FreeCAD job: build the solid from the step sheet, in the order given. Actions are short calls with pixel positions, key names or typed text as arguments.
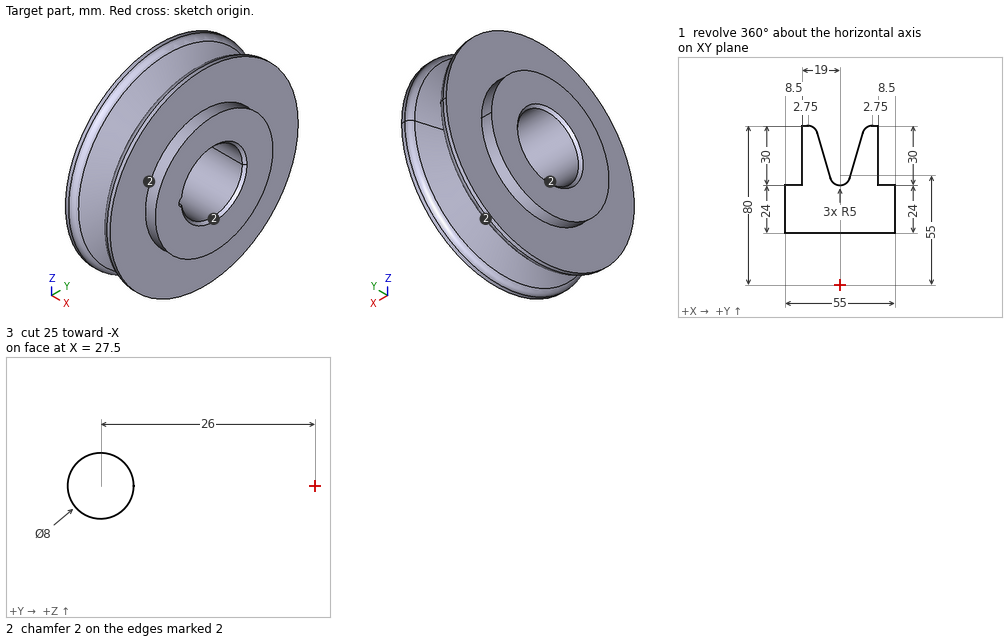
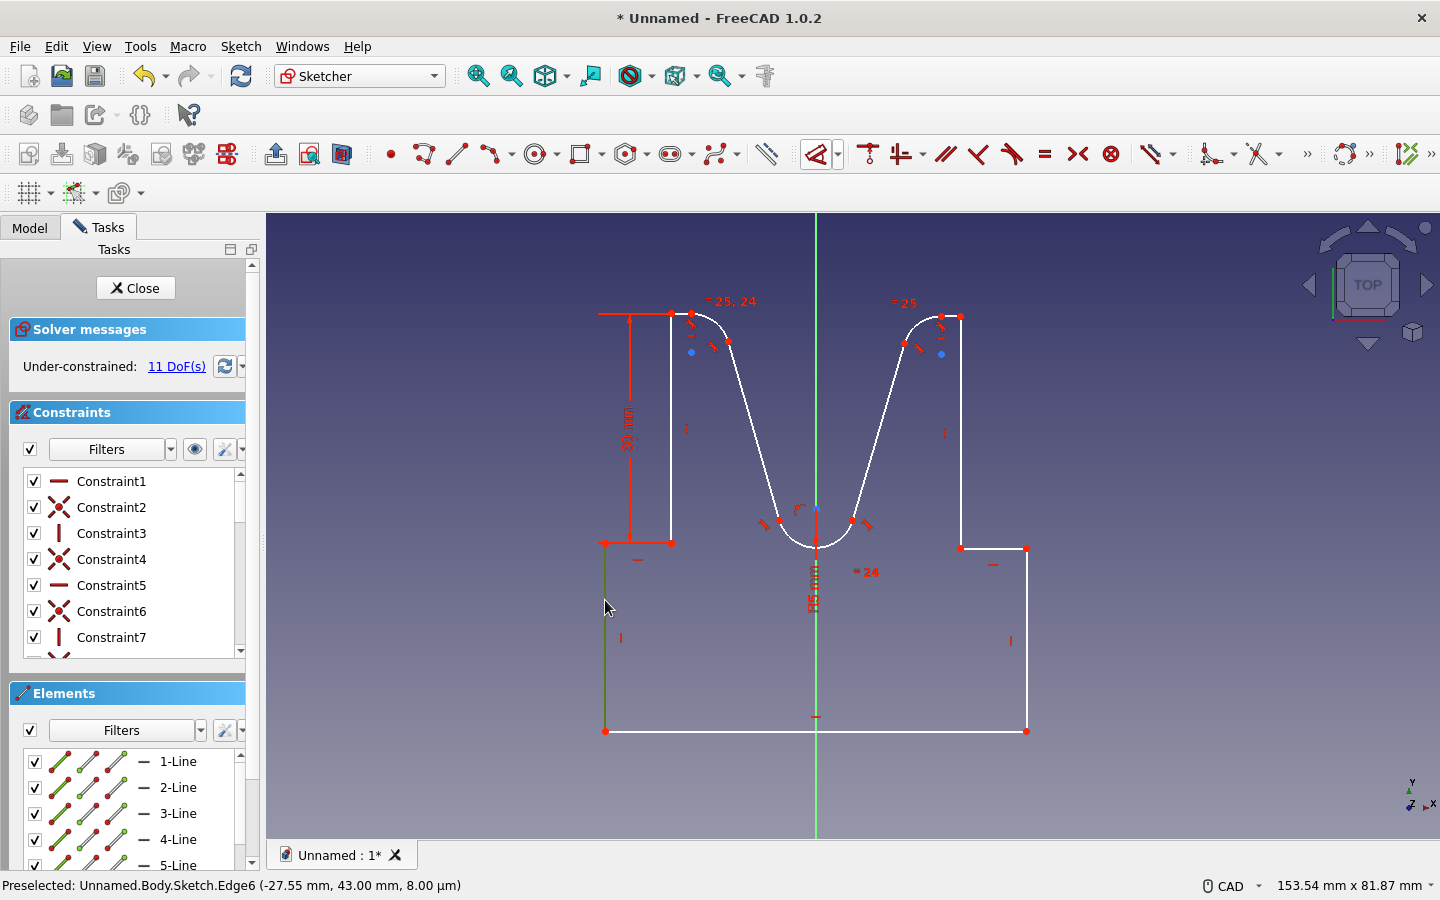
click(838, 154)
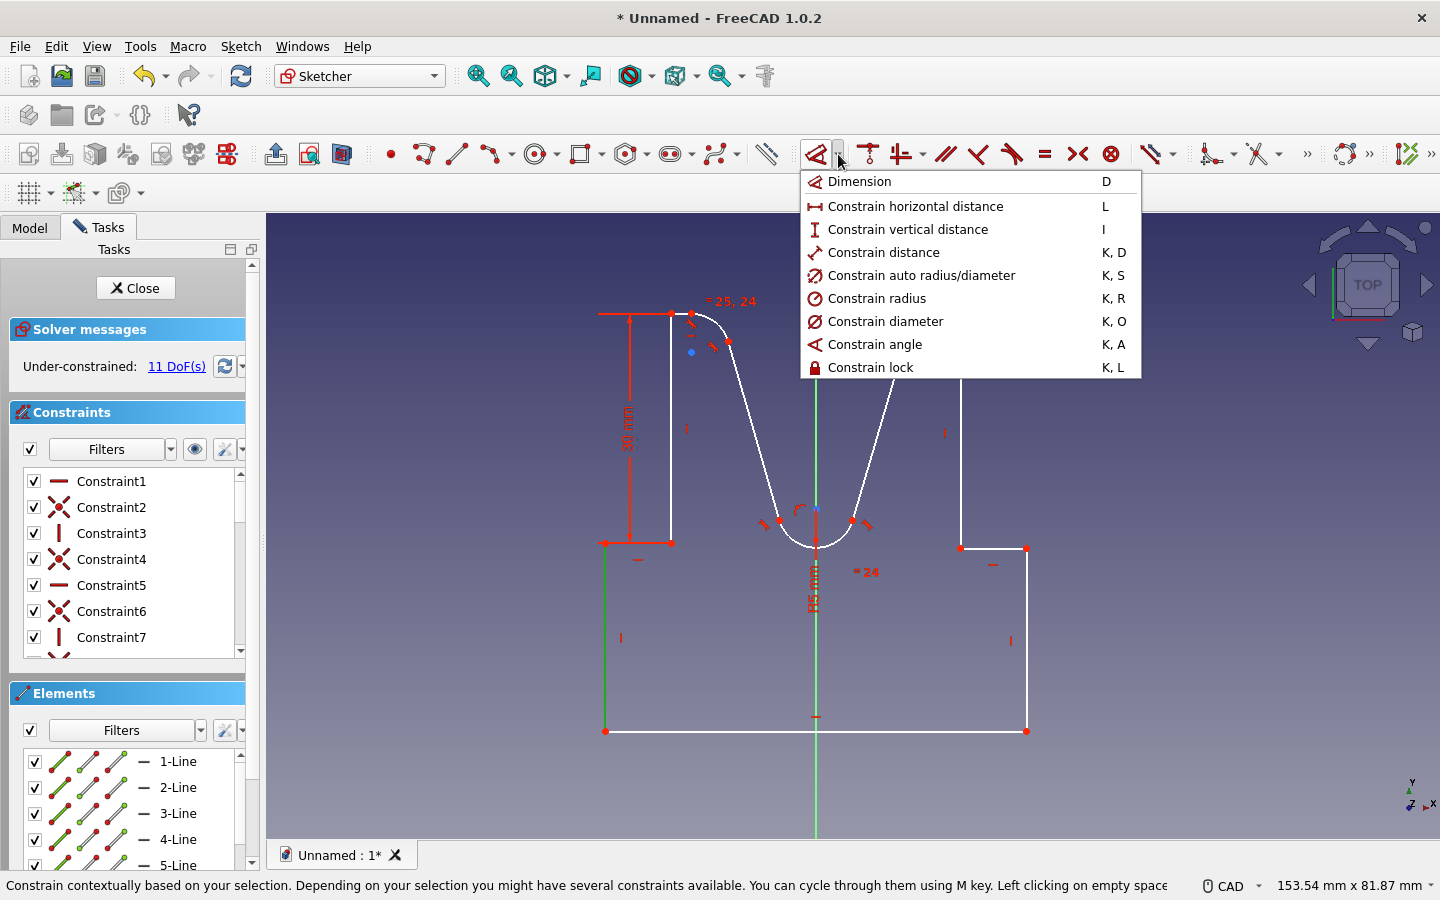
click(971, 230)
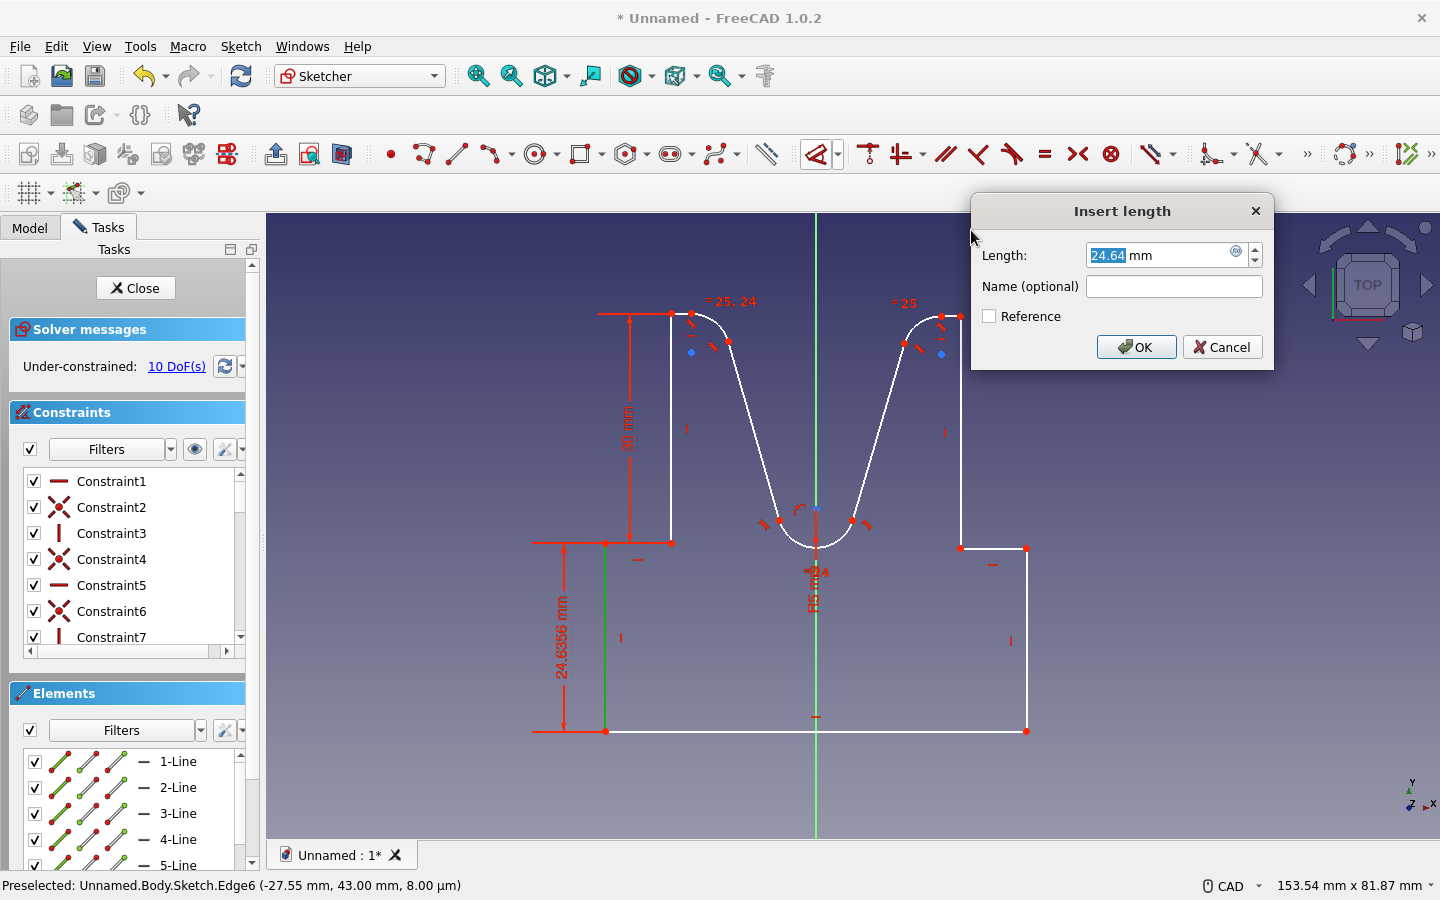
text(24)
key(Return)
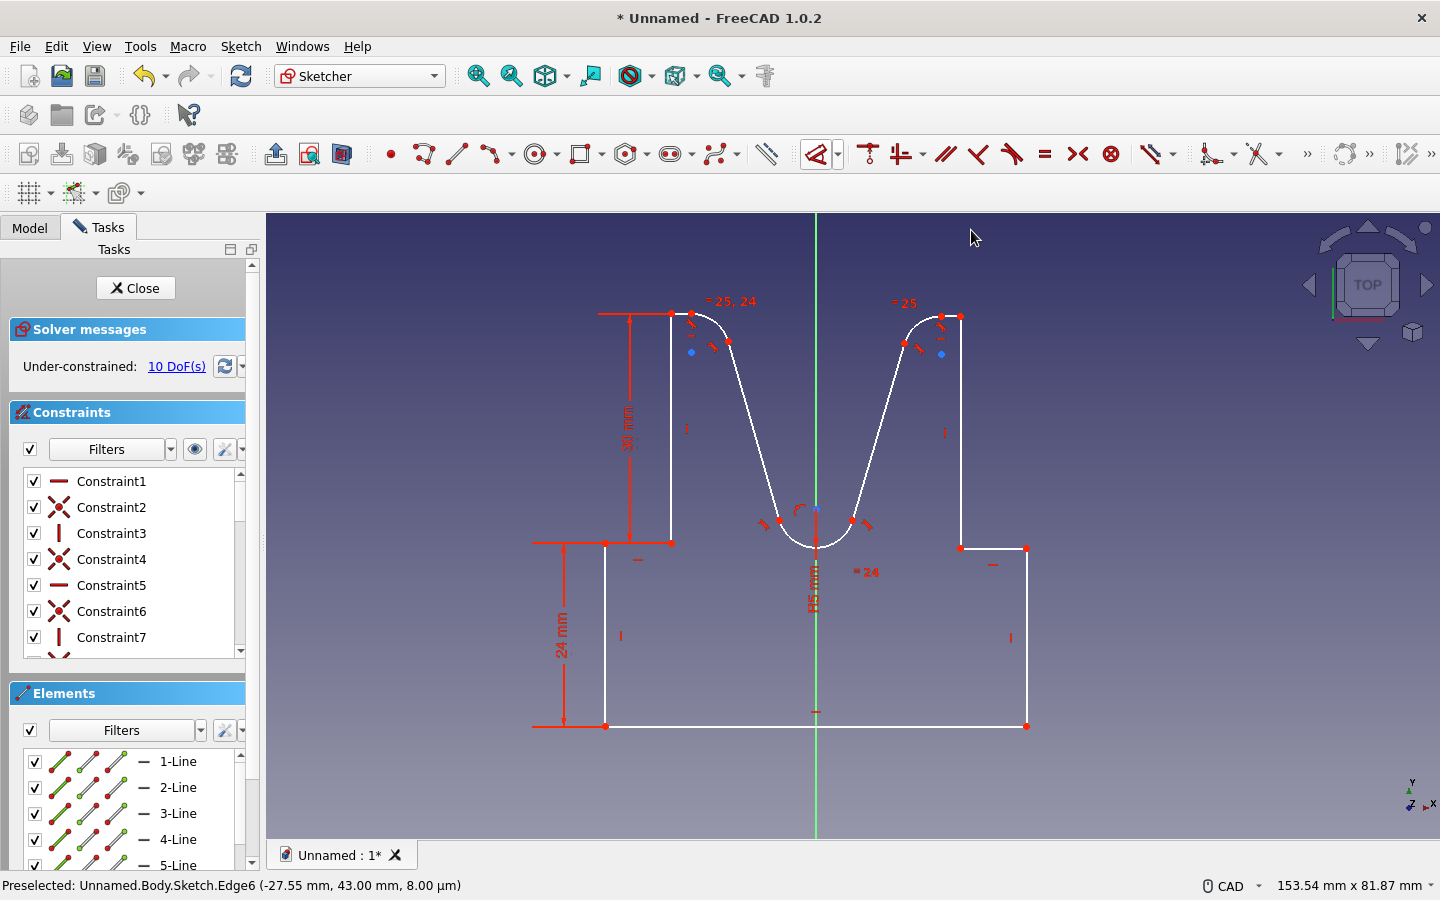
click(732, 727)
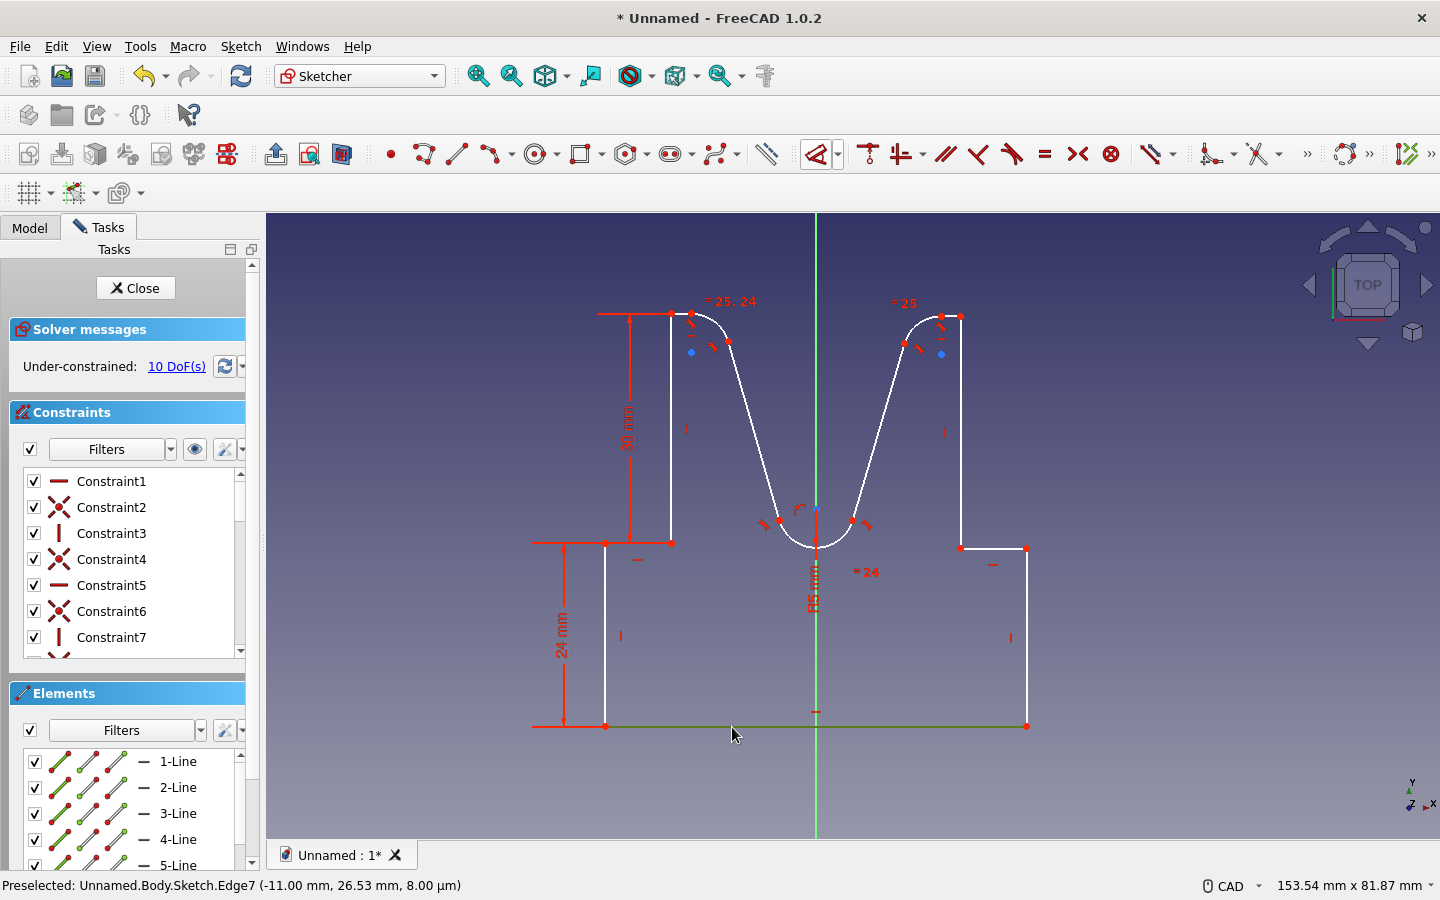
key(l)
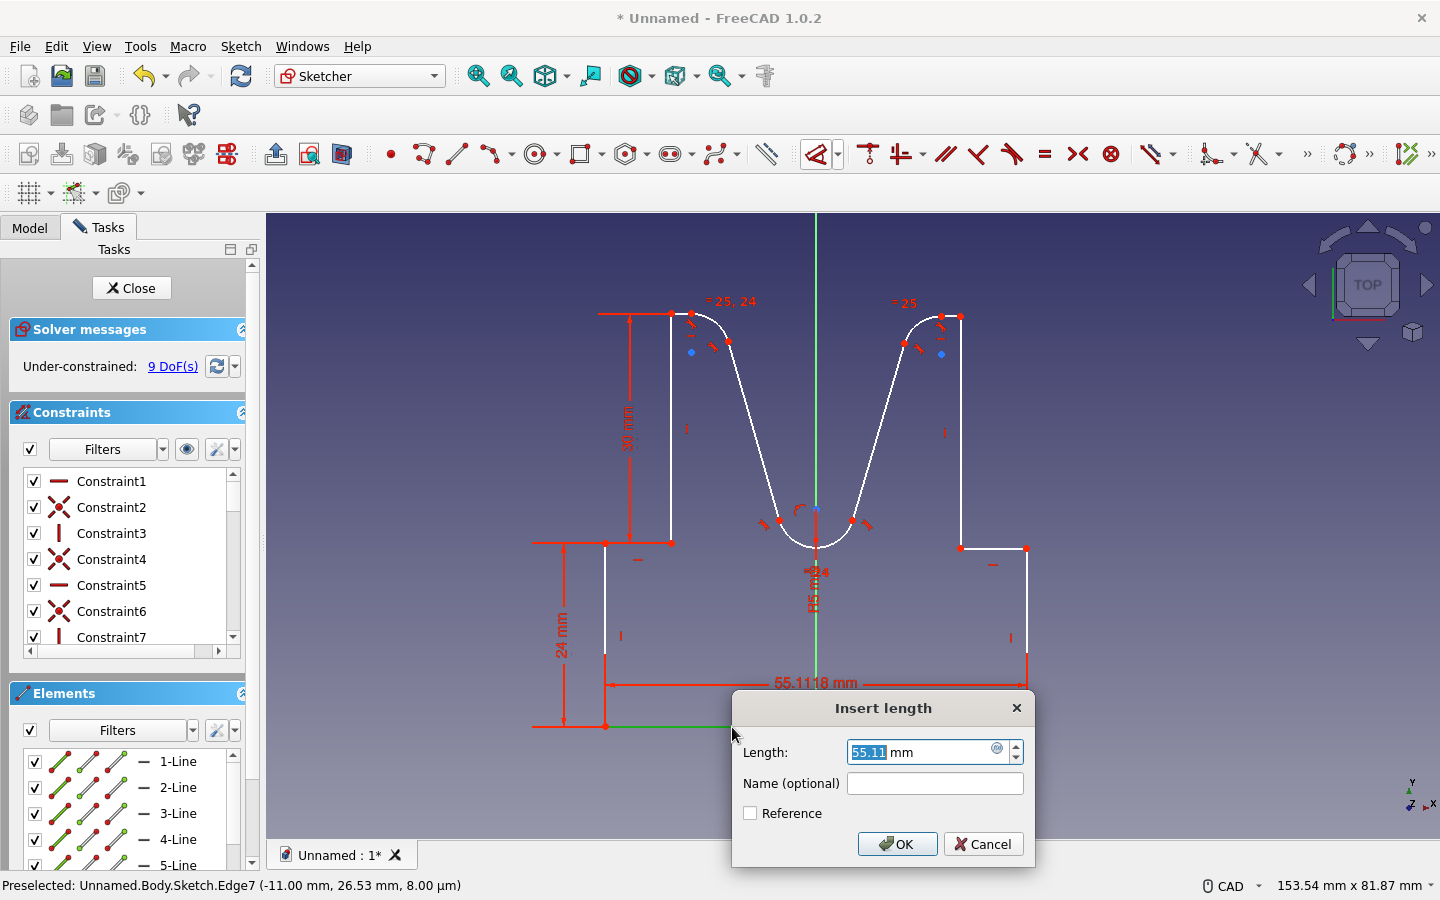
text(55)
key(Return)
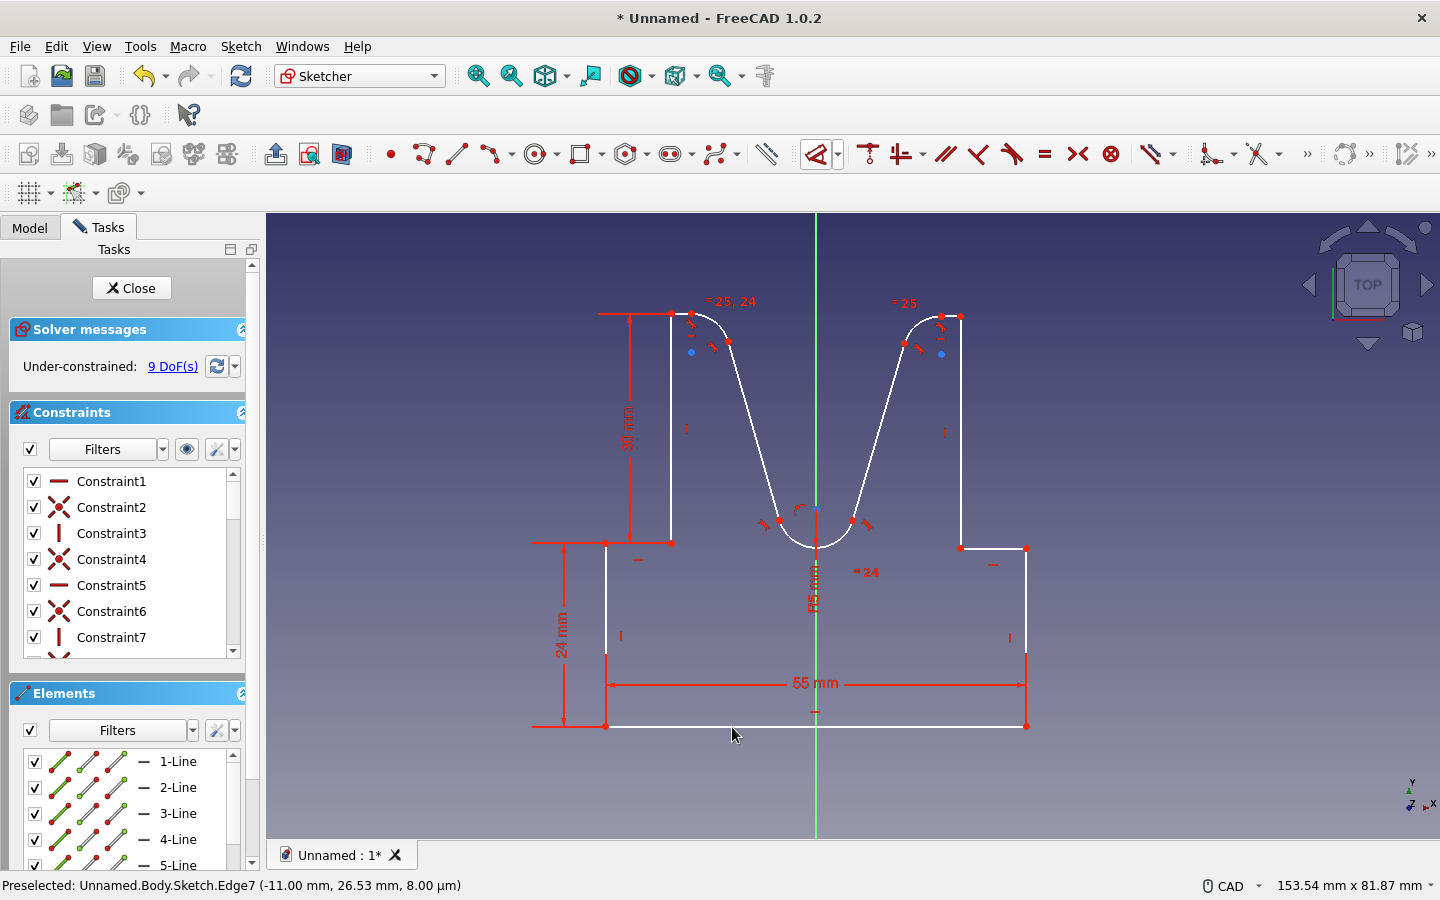
click(1026, 673)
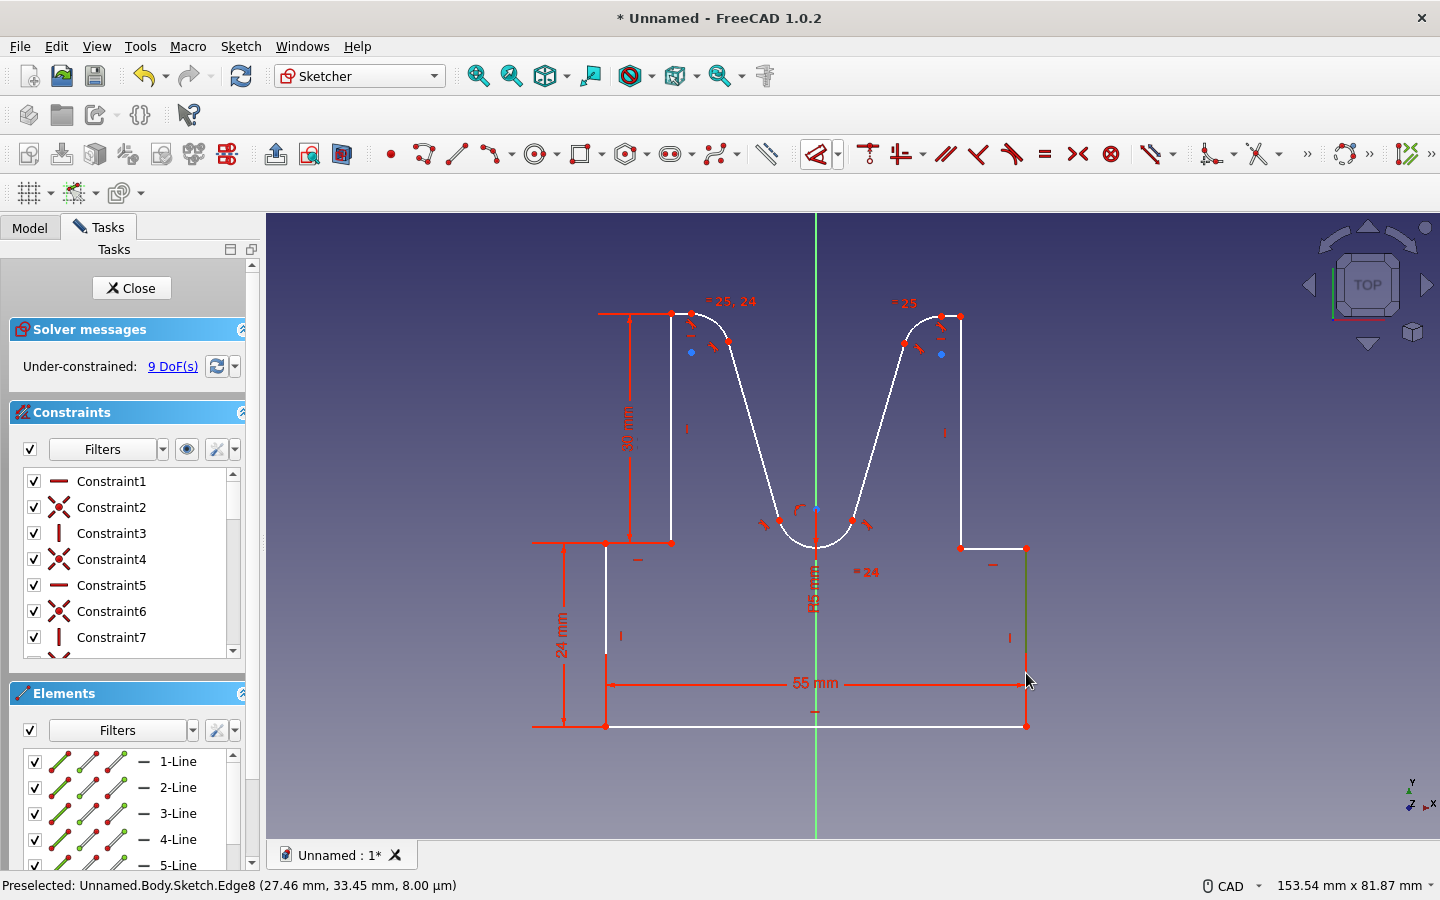
key(i)